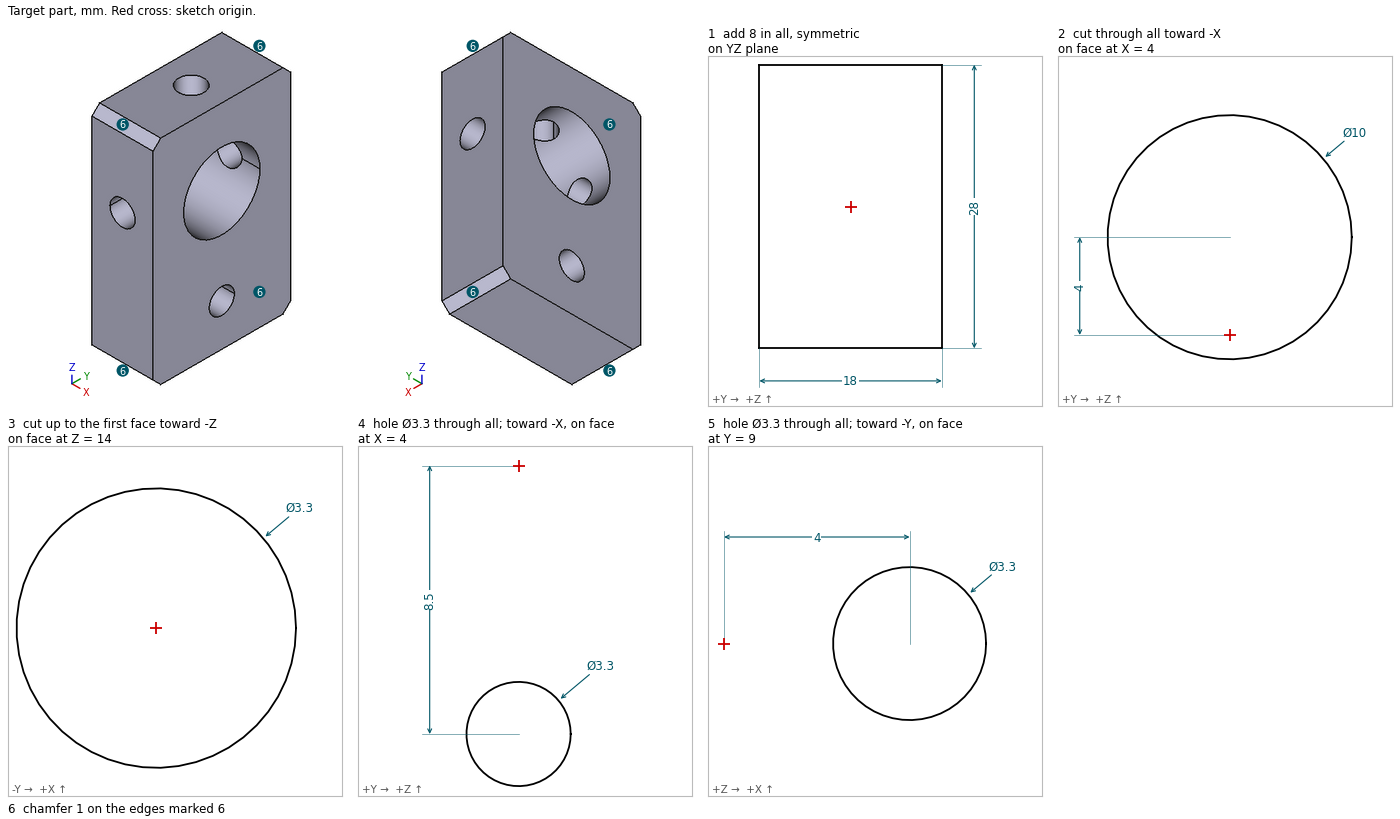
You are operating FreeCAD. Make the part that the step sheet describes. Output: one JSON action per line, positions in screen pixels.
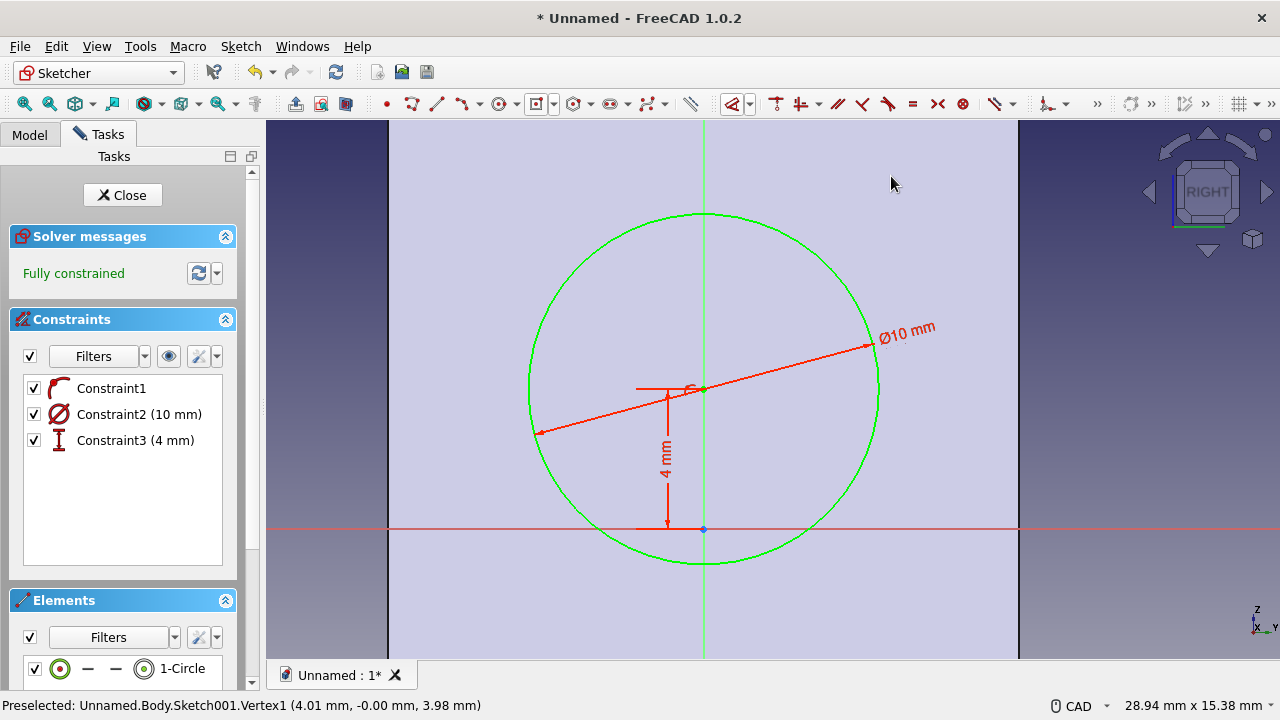
{"action": "left_click", "coordinate": [123, 195]}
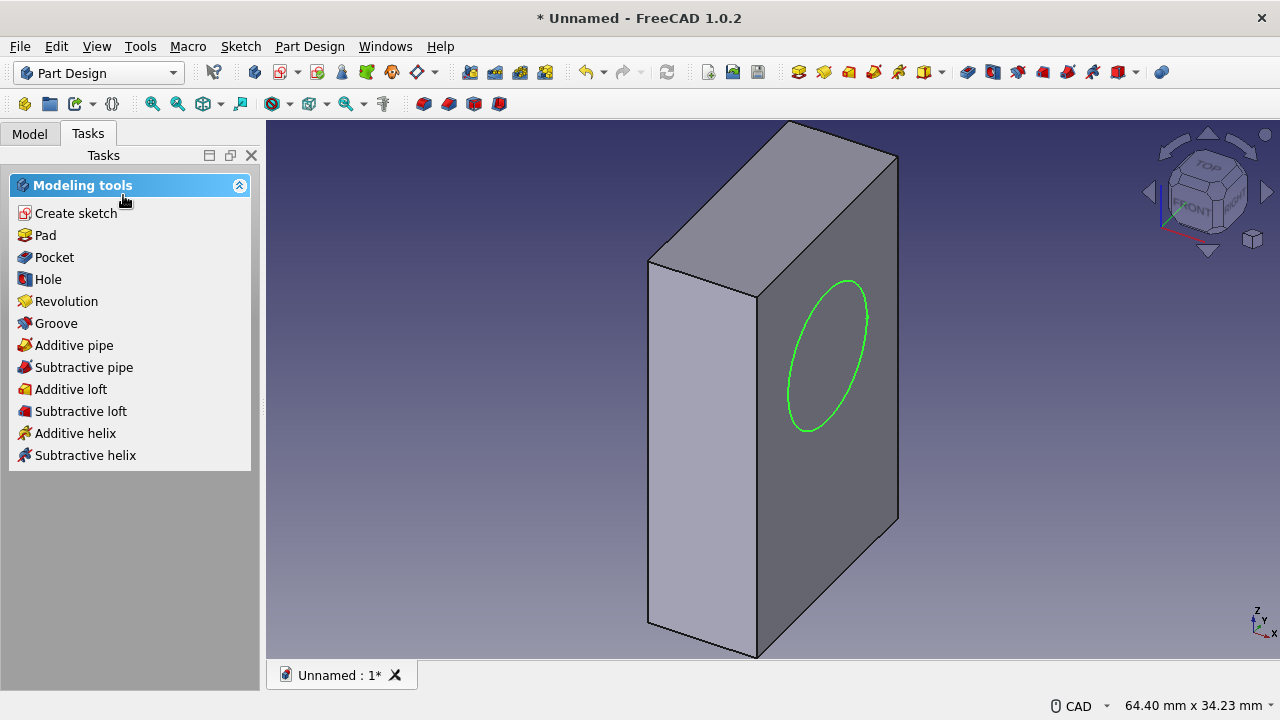
{"action": "left_click", "coordinate": [968, 72]}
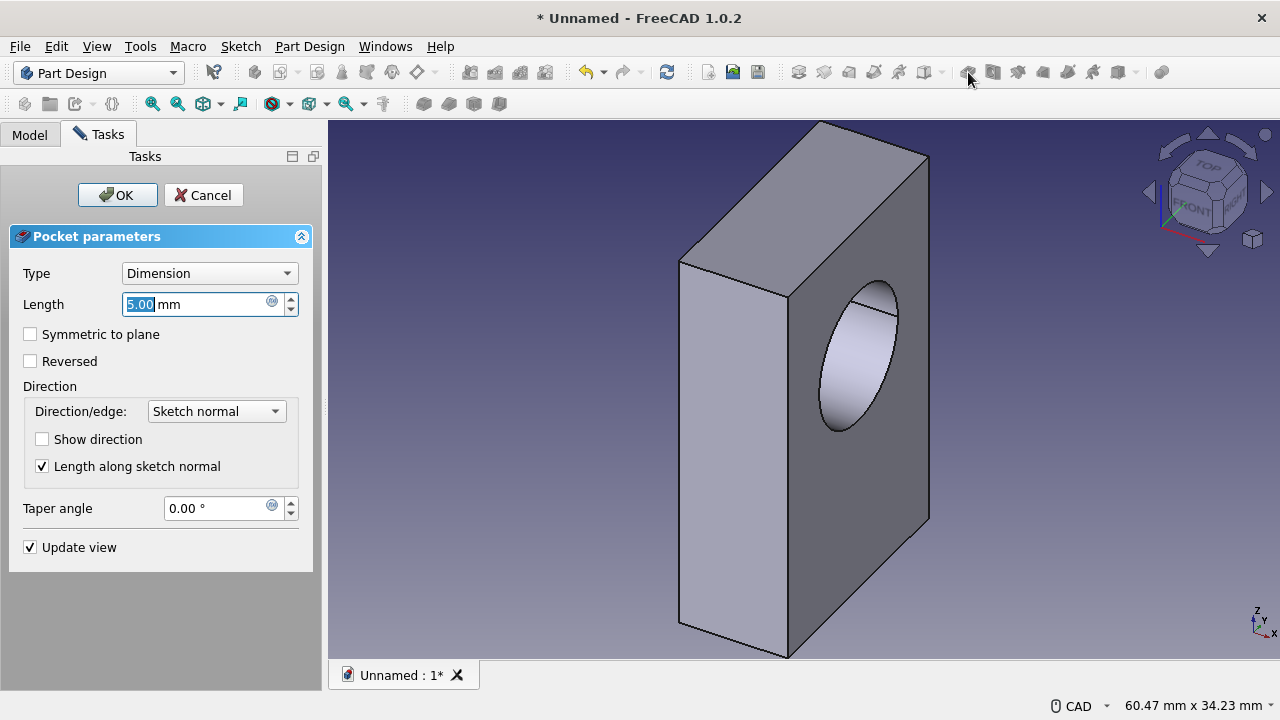
{"action": "left_click", "coordinate": [210, 274]}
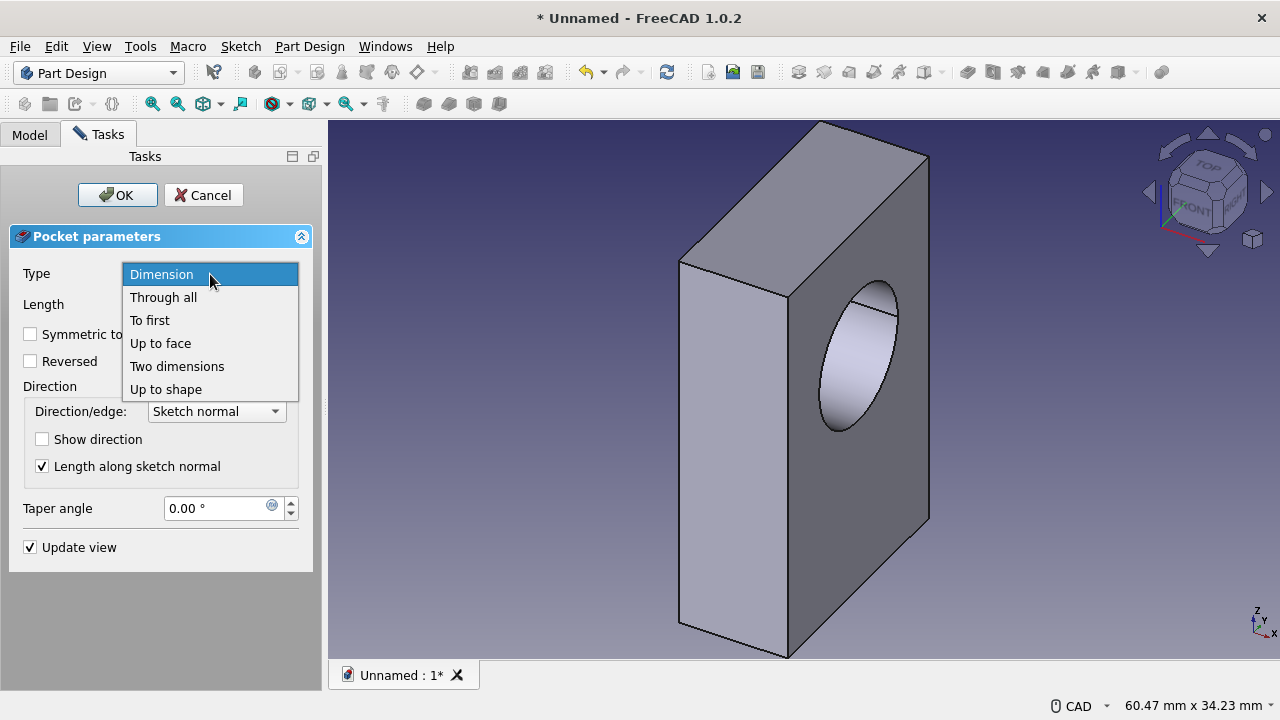
{"action": "left_click", "coordinate": [208, 298]}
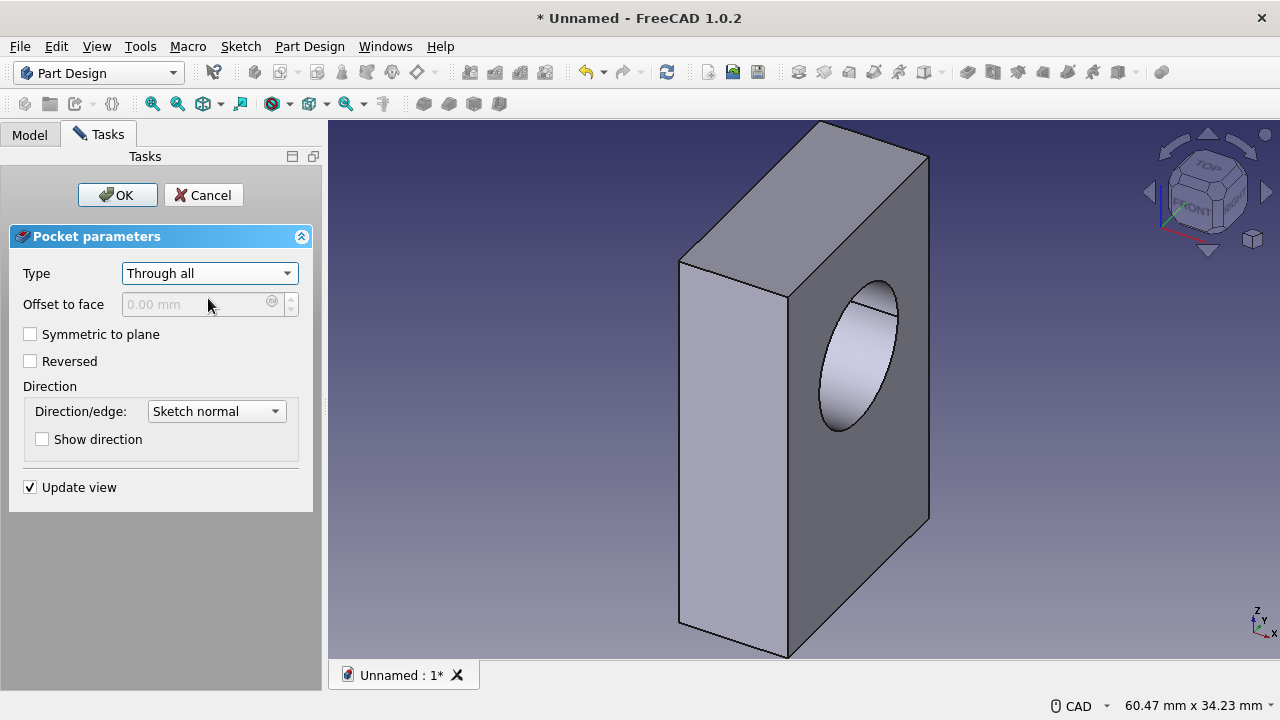
{"action": "left_click", "coordinate": [118, 195]}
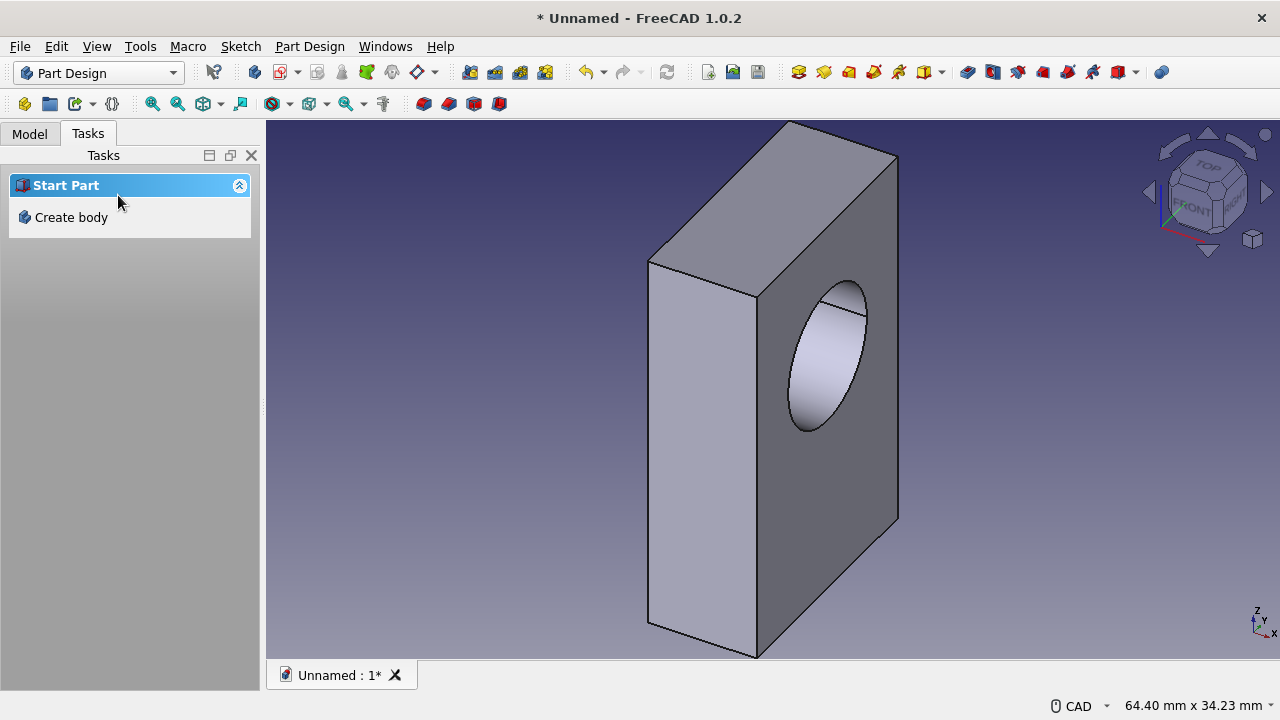
{"action": "left_click", "coordinate": [153, 104]}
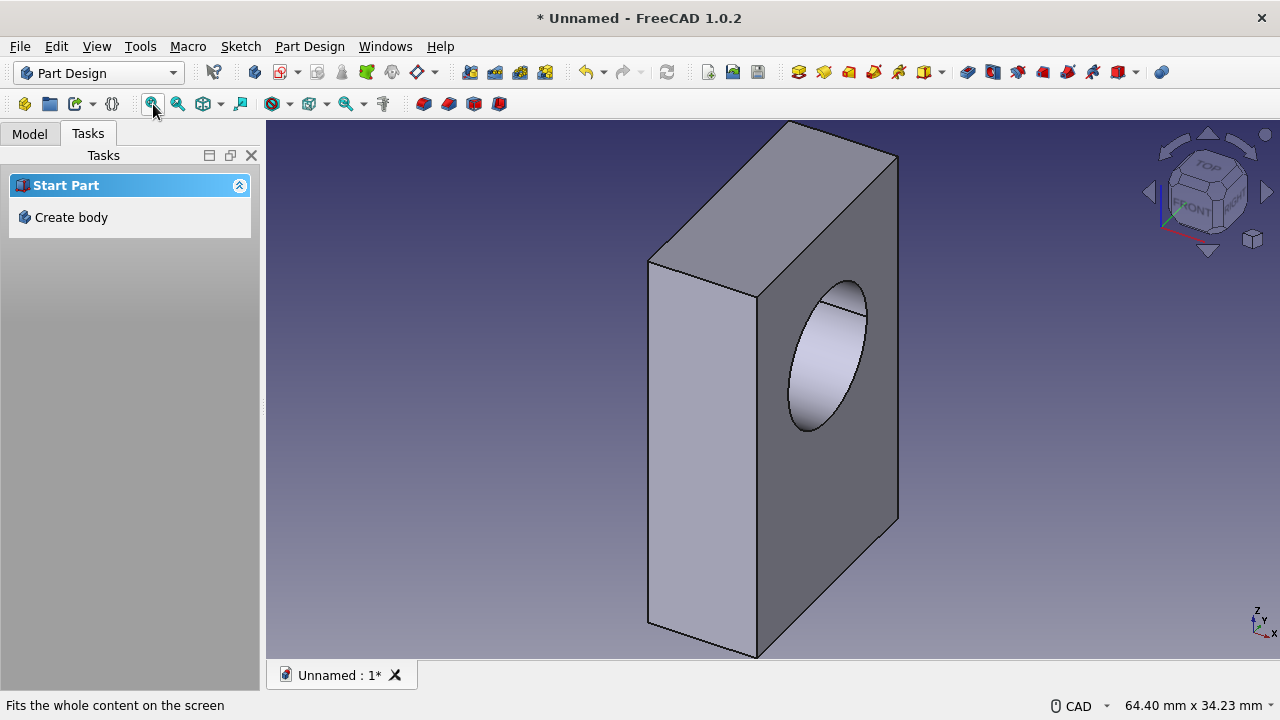
{"action": "left_click", "coordinate": [793, 188]}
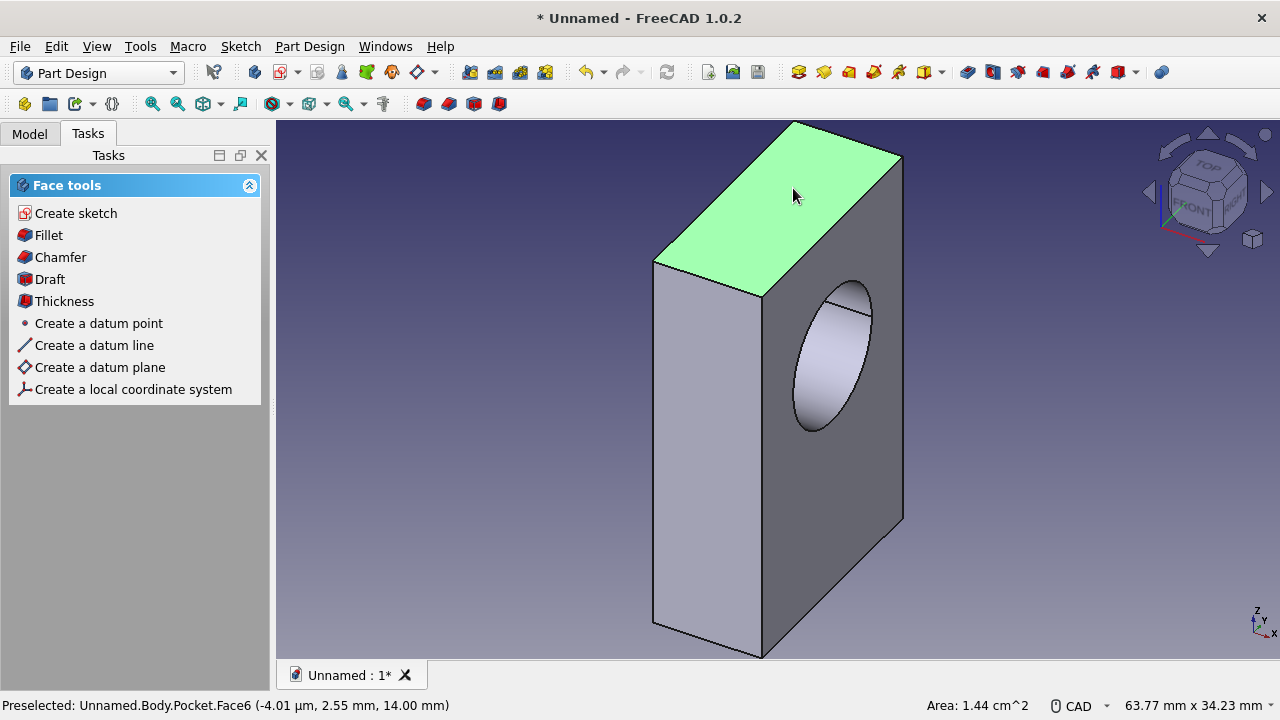
{"action": "left_click", "coordinate": [280, 72]}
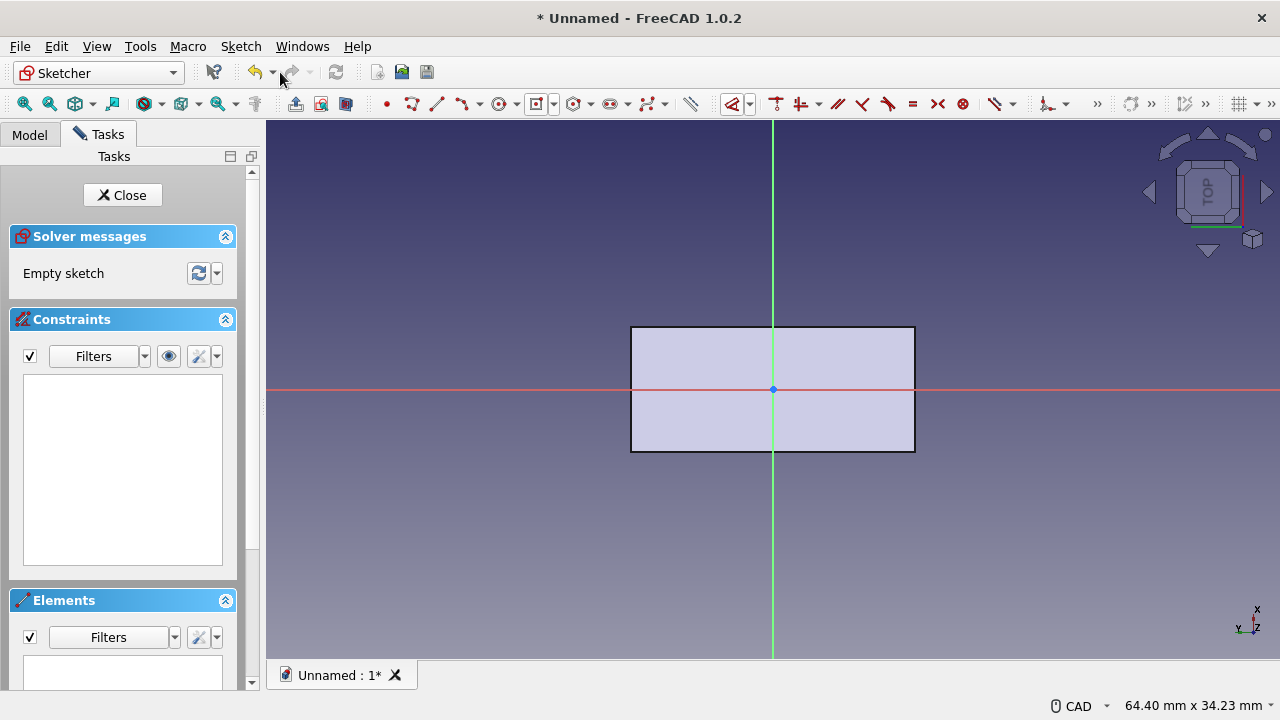
{"action": "scroll", "coordinate": [787, 390], "scroll_direction": "up", "scroll_amount": 9}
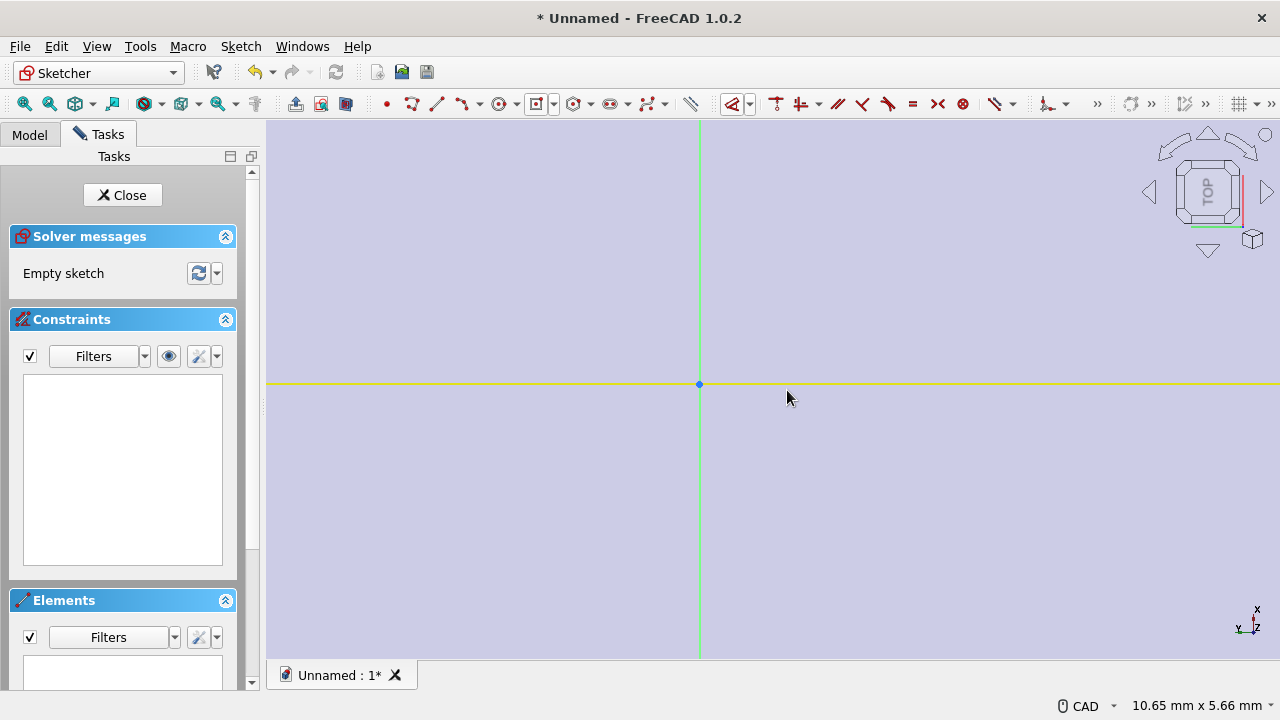
{"action": "left_click", "coordinate": [498, 104]}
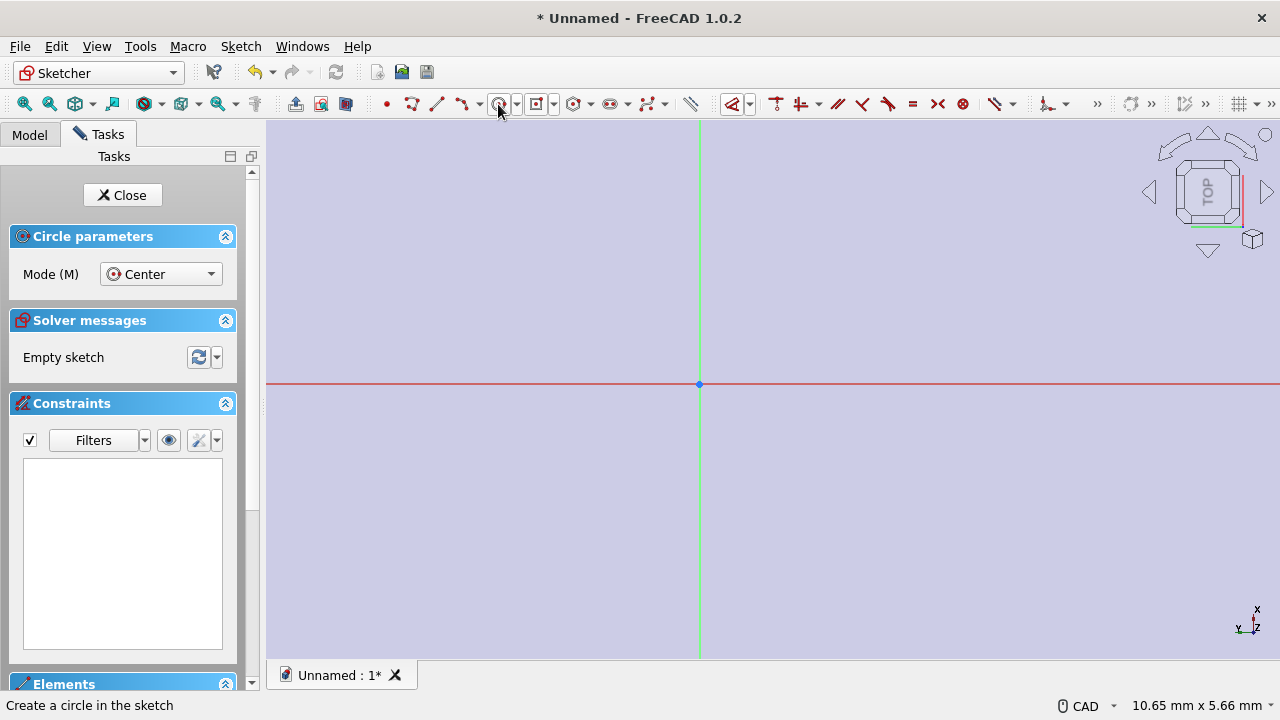
{"action": "left_click", "coordinate": [700, 384]}
{"action": "left_click", "coordinate": [811, 273]}
{"action": "key", "text": "Escape"}